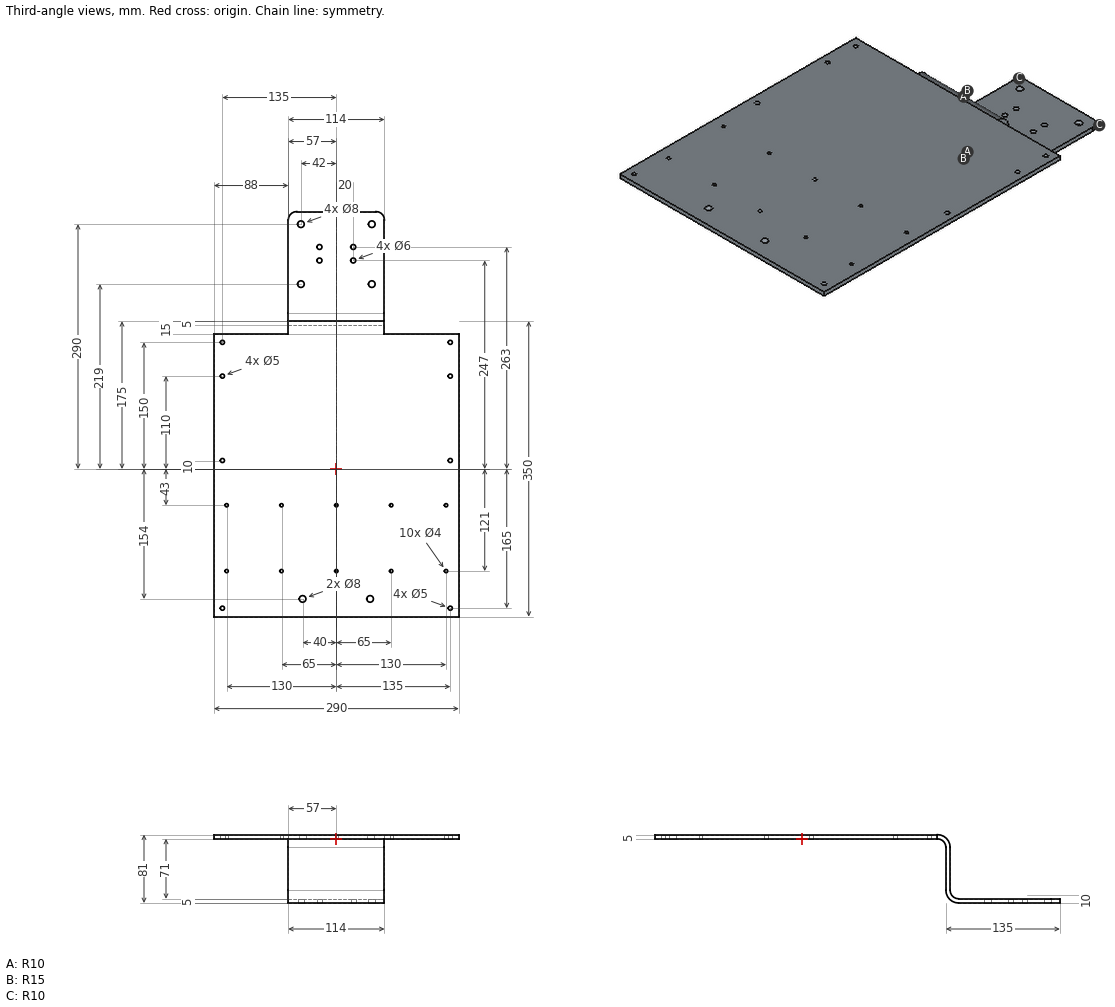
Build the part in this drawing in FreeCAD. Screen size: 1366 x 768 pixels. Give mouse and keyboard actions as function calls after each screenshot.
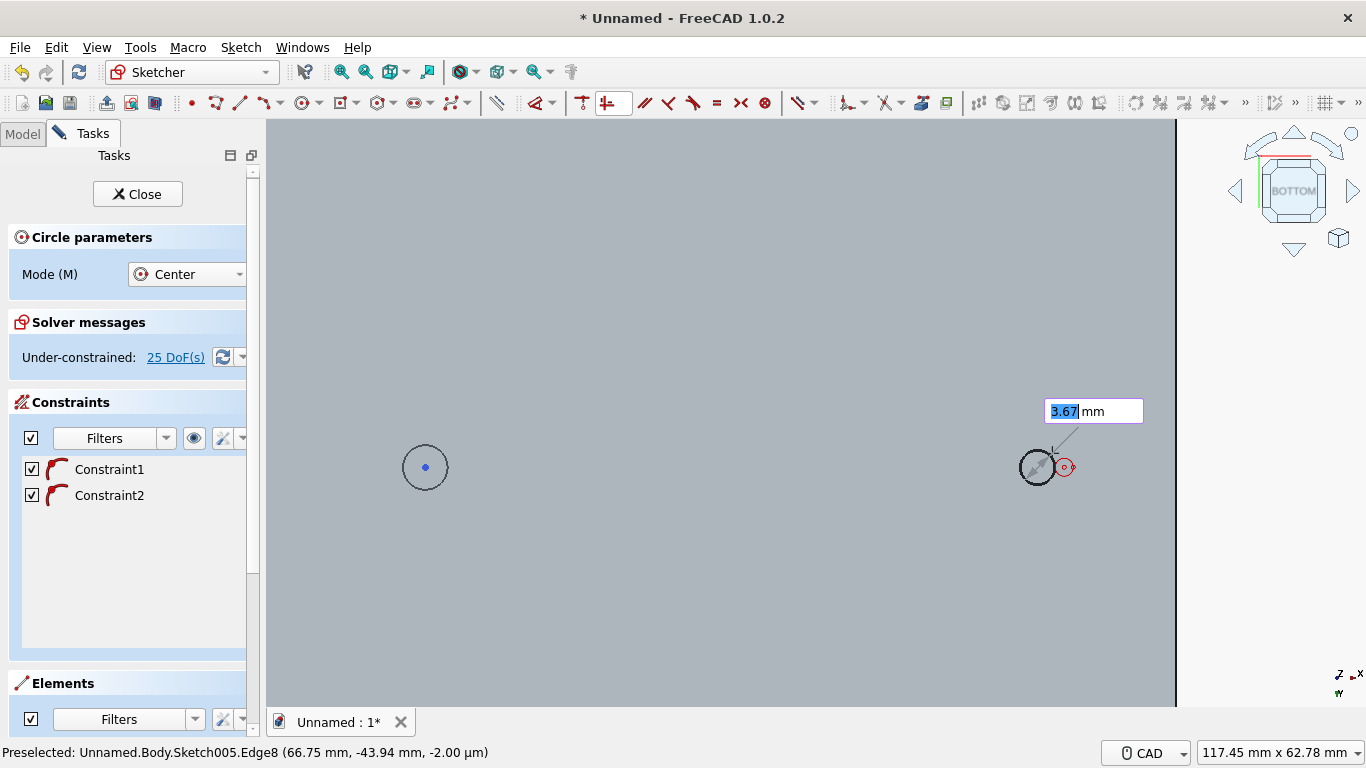
click(1049, 450)
key(Escape)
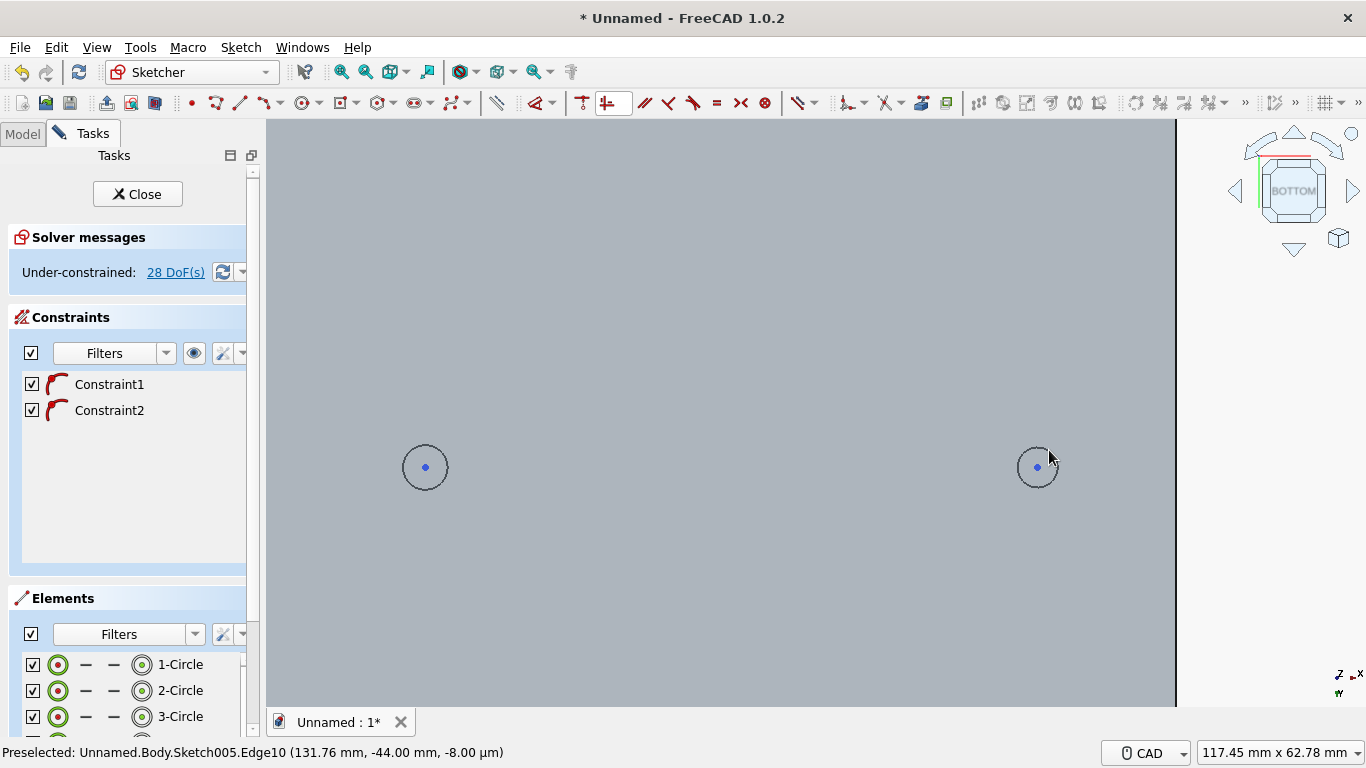
scroll(1052, 453, down, 7)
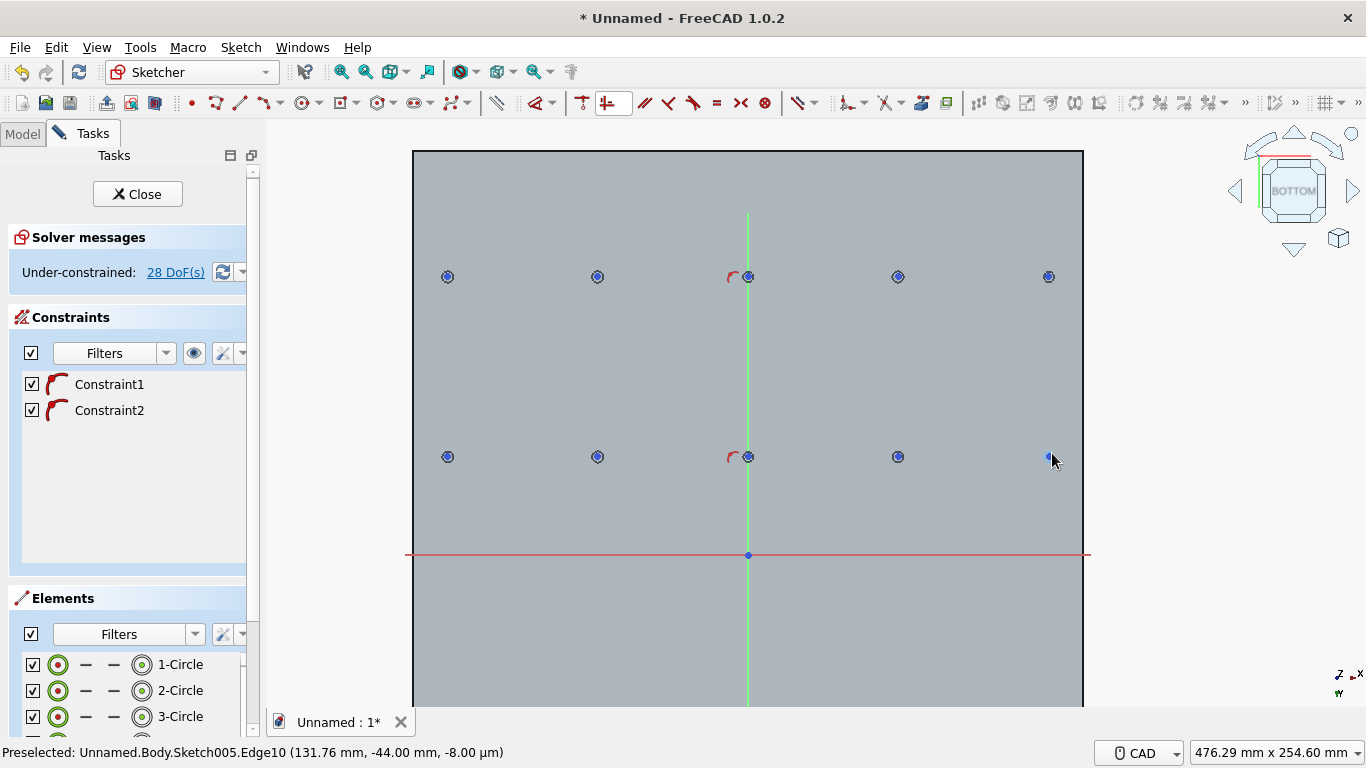
scroll(1053, 273, up, 5)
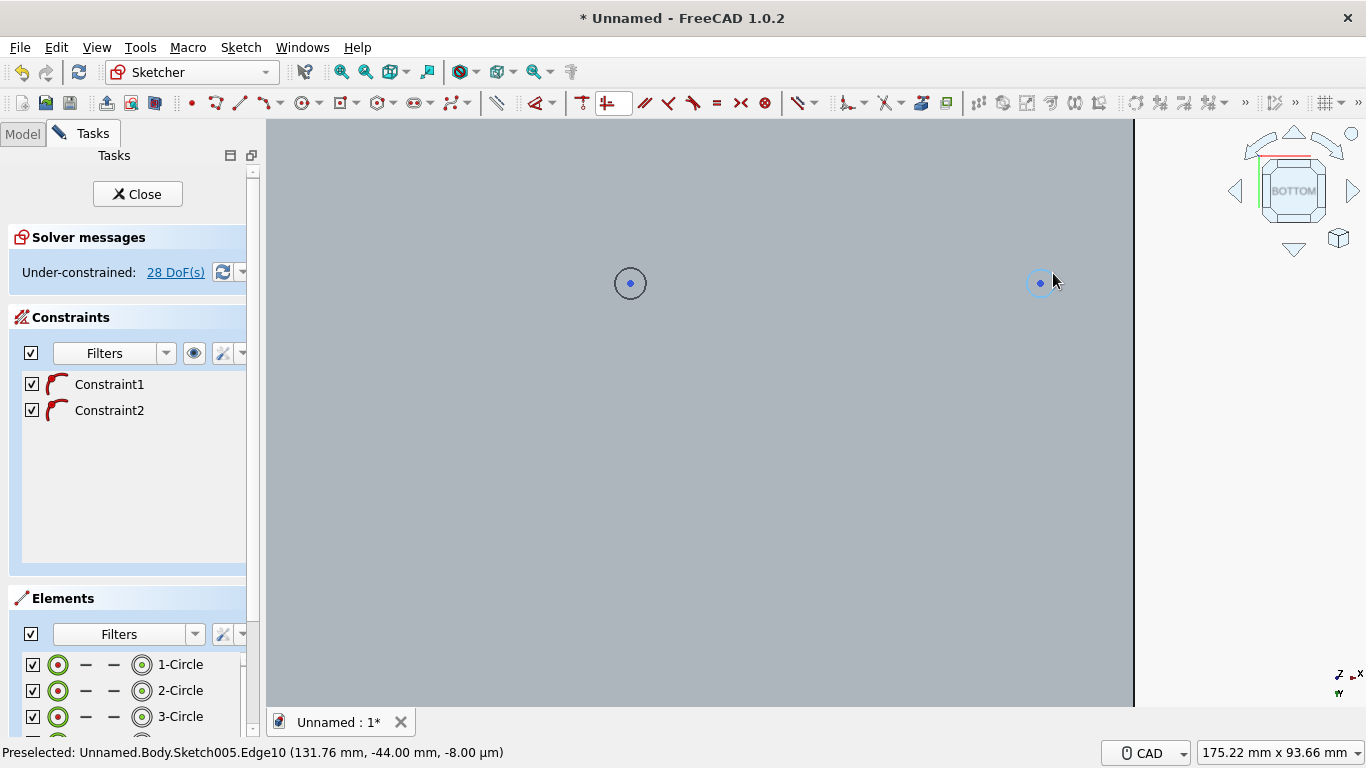
click(1051, 274)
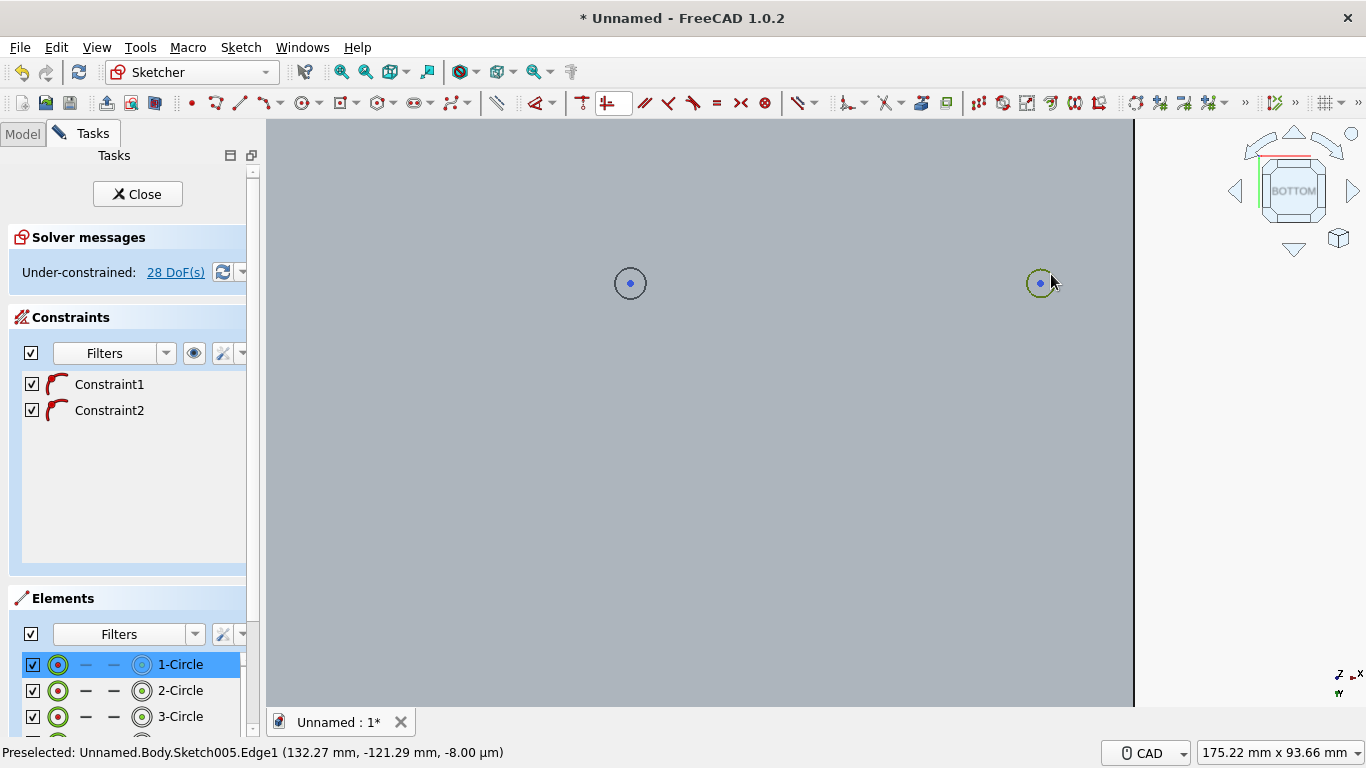
click(641, 272)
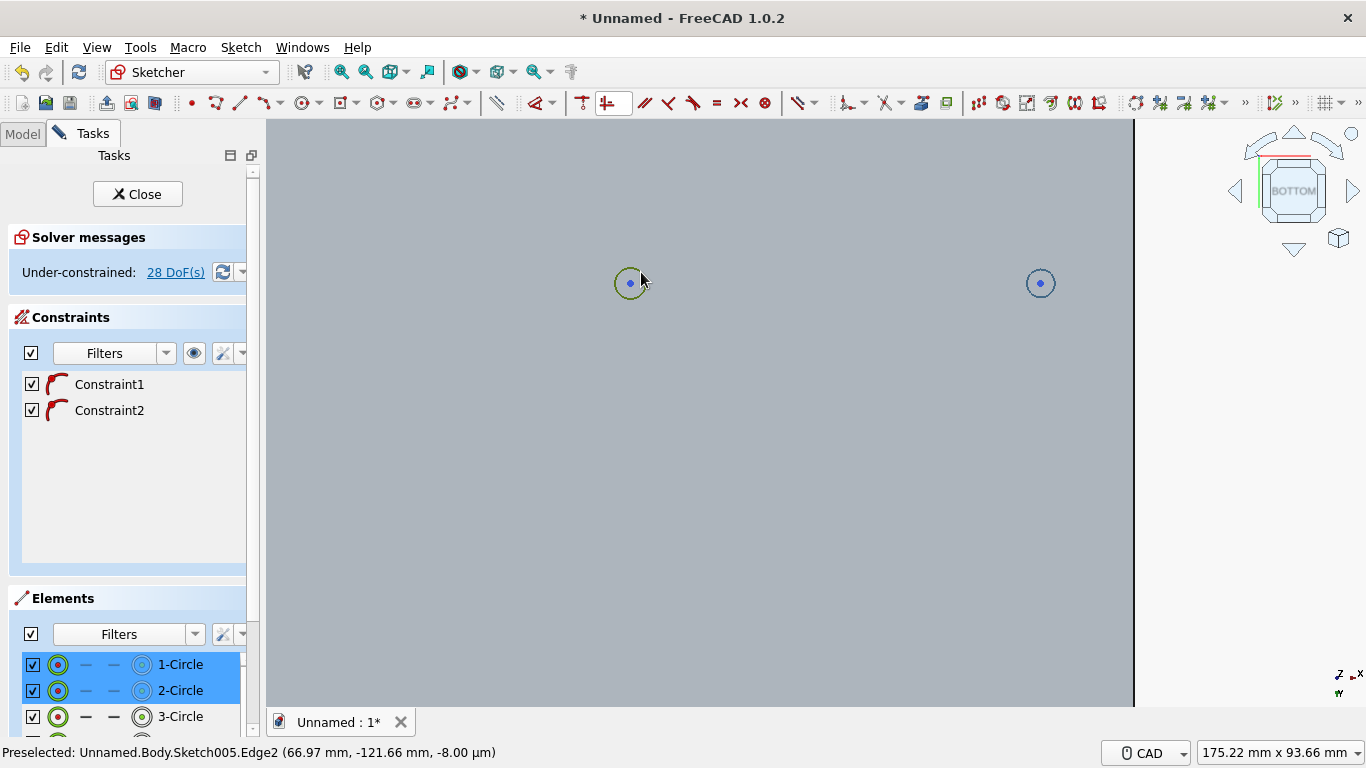
scroll(1052, 273, down, 5)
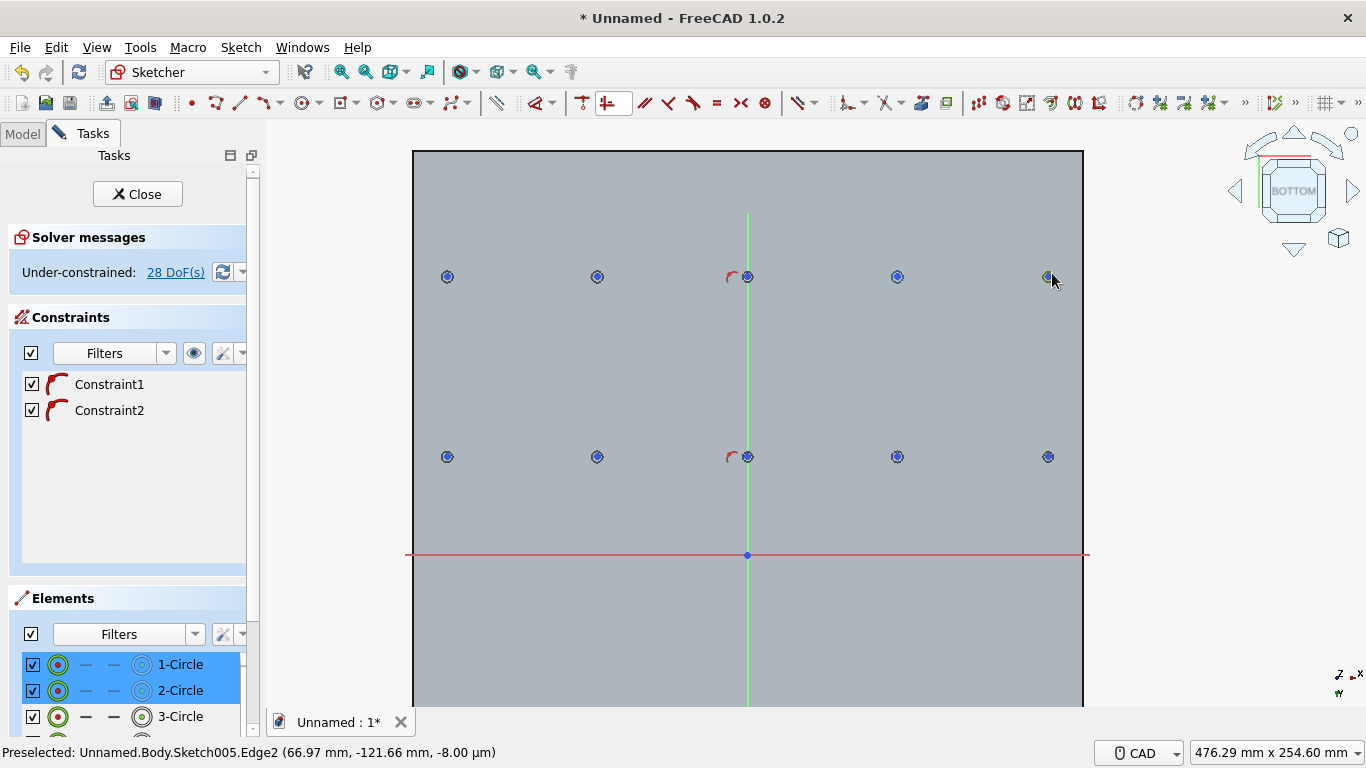
scroll(751, 273, up, 7)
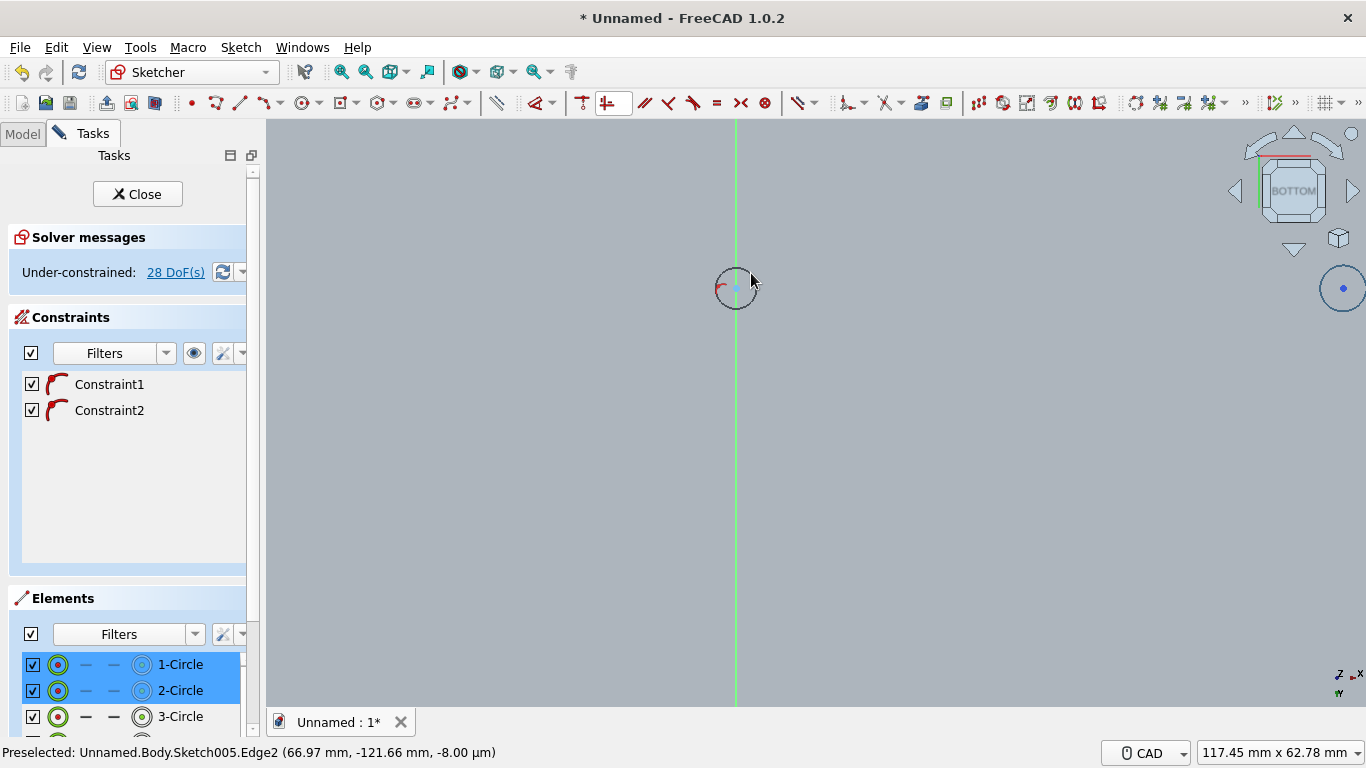
click(751, 274)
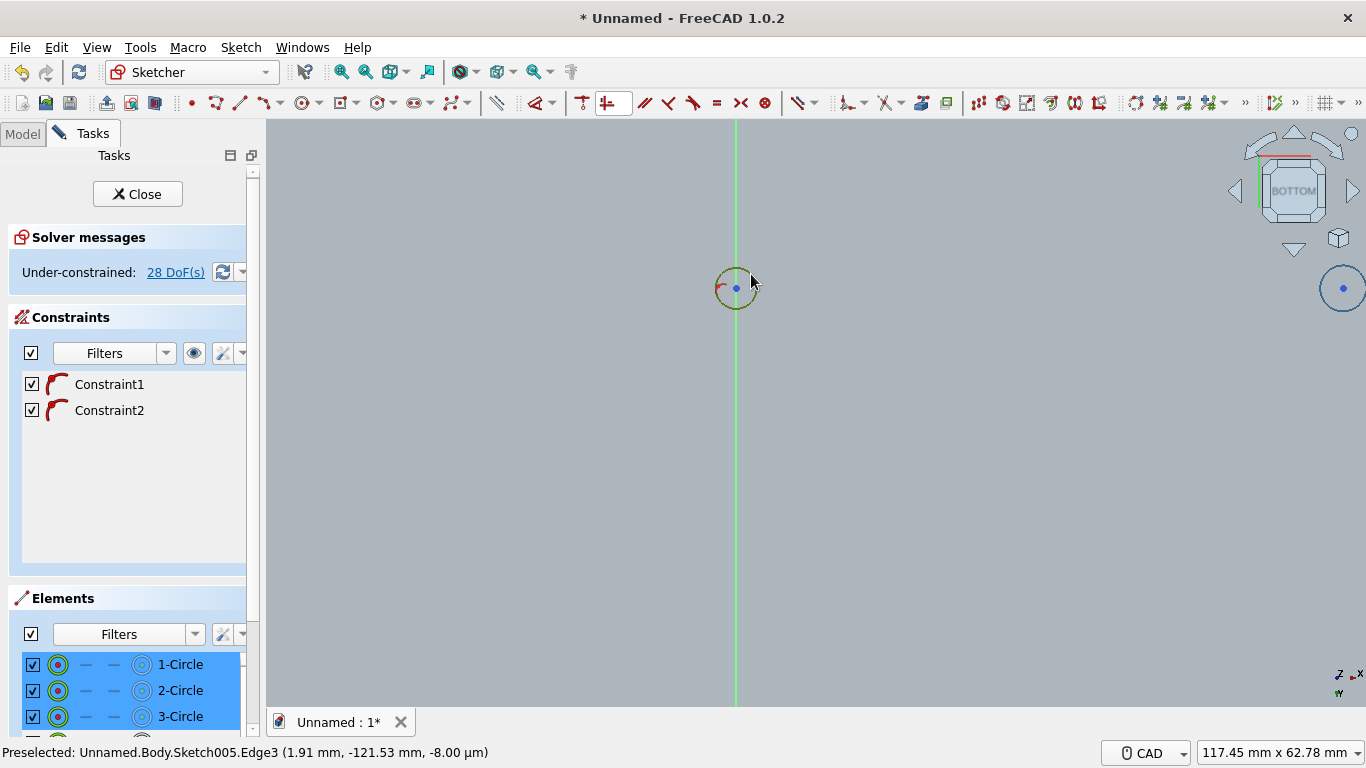
scroll(751, 273, down, 7)